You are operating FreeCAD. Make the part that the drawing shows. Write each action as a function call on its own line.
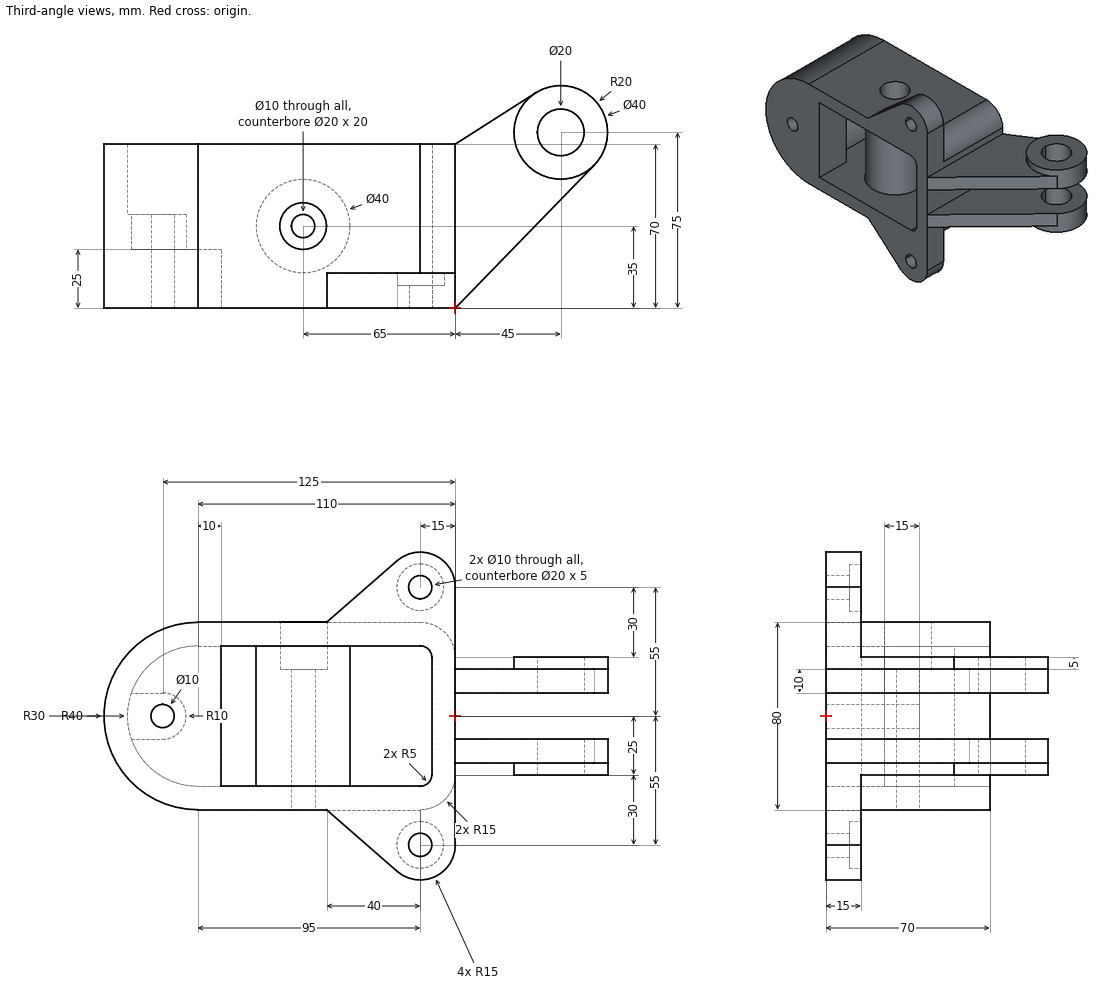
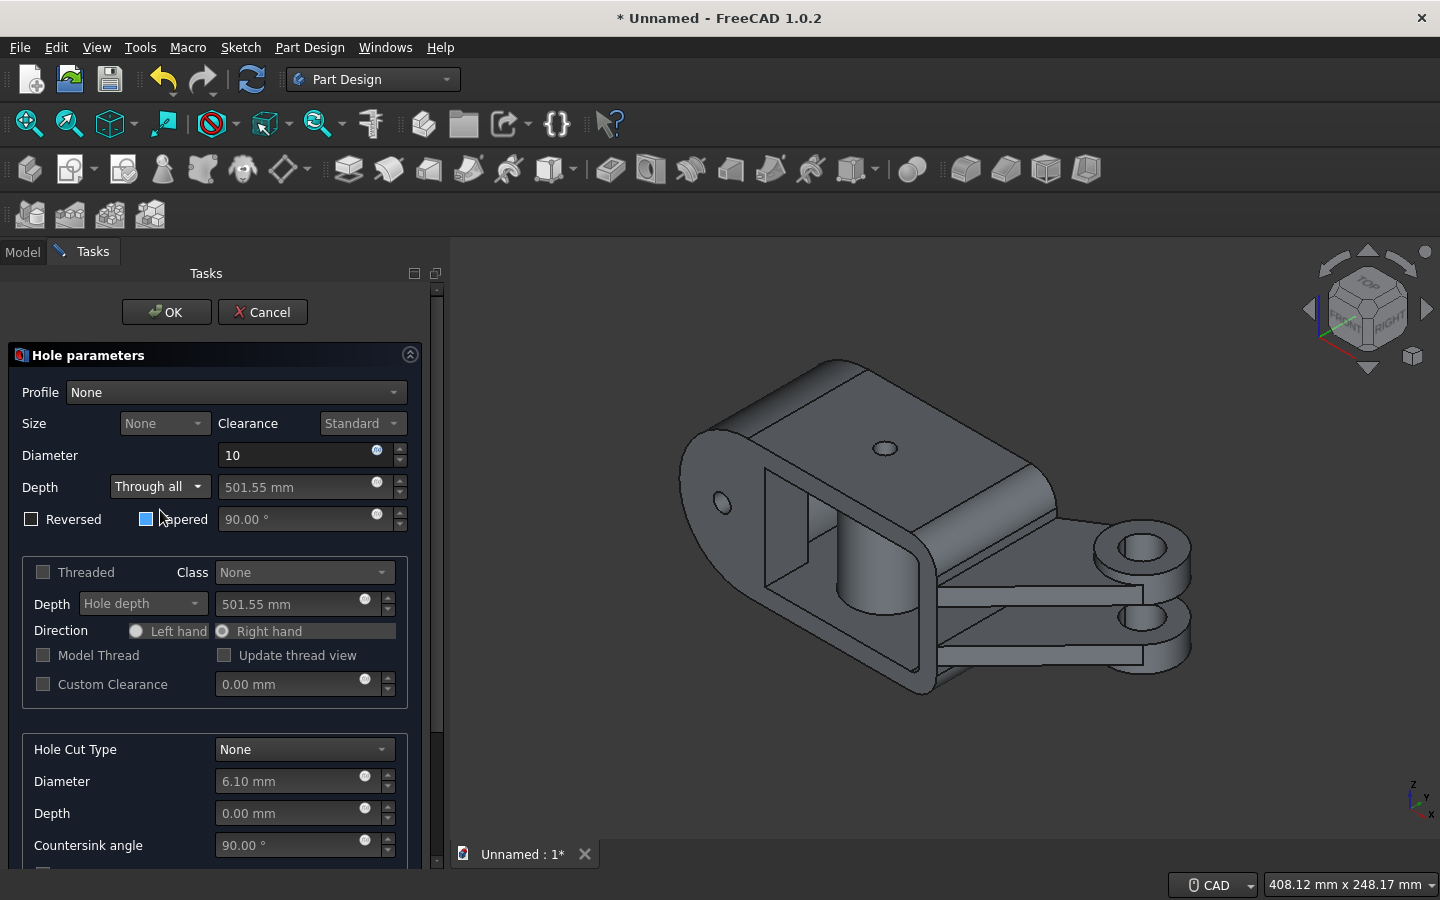
click(306, 750)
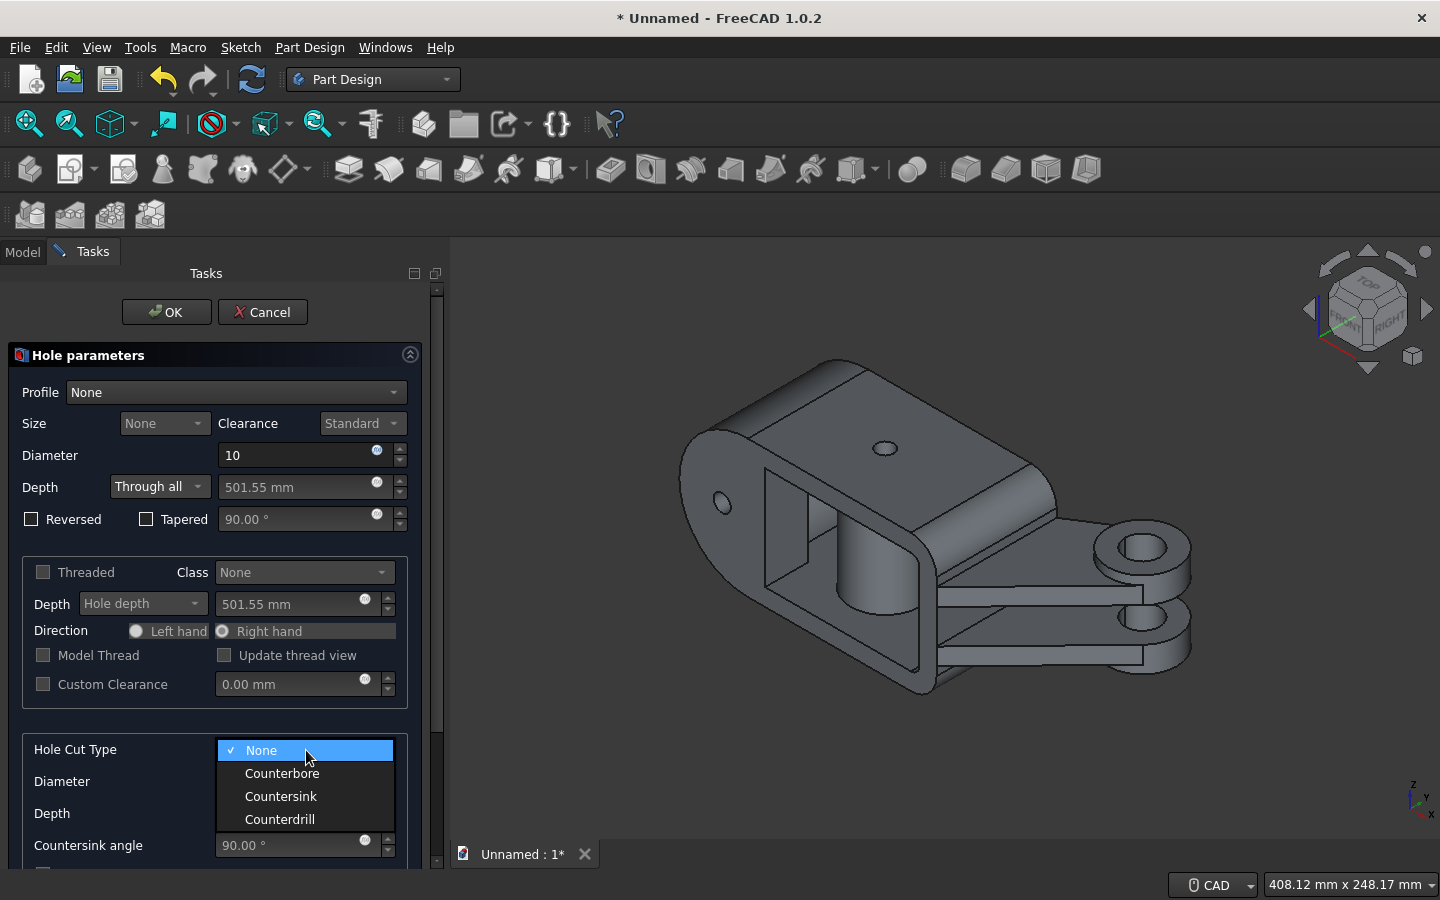
click(304, 774)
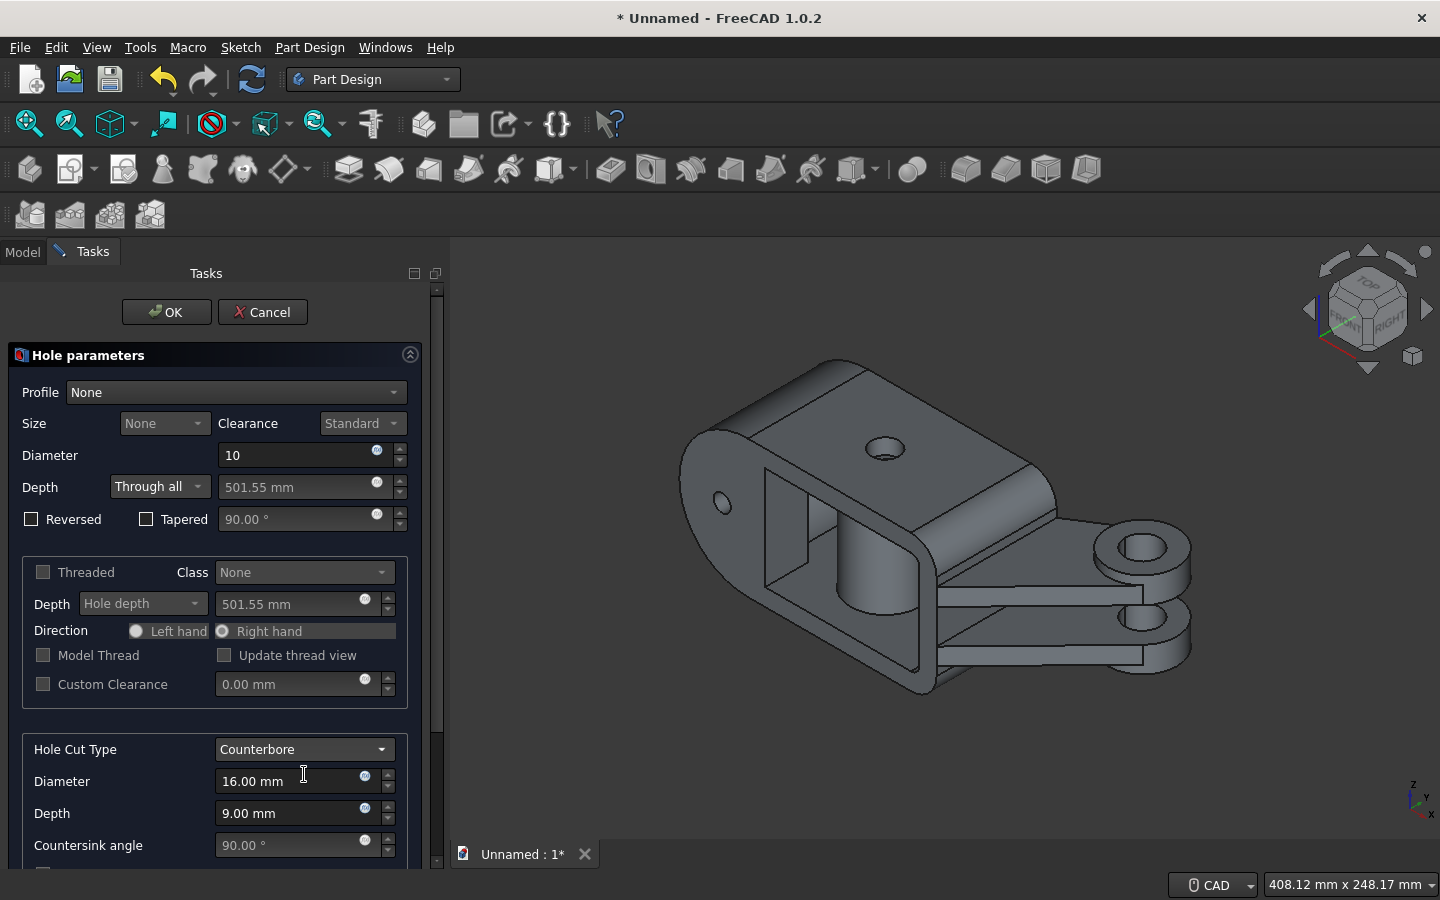
triple_click(298, 781)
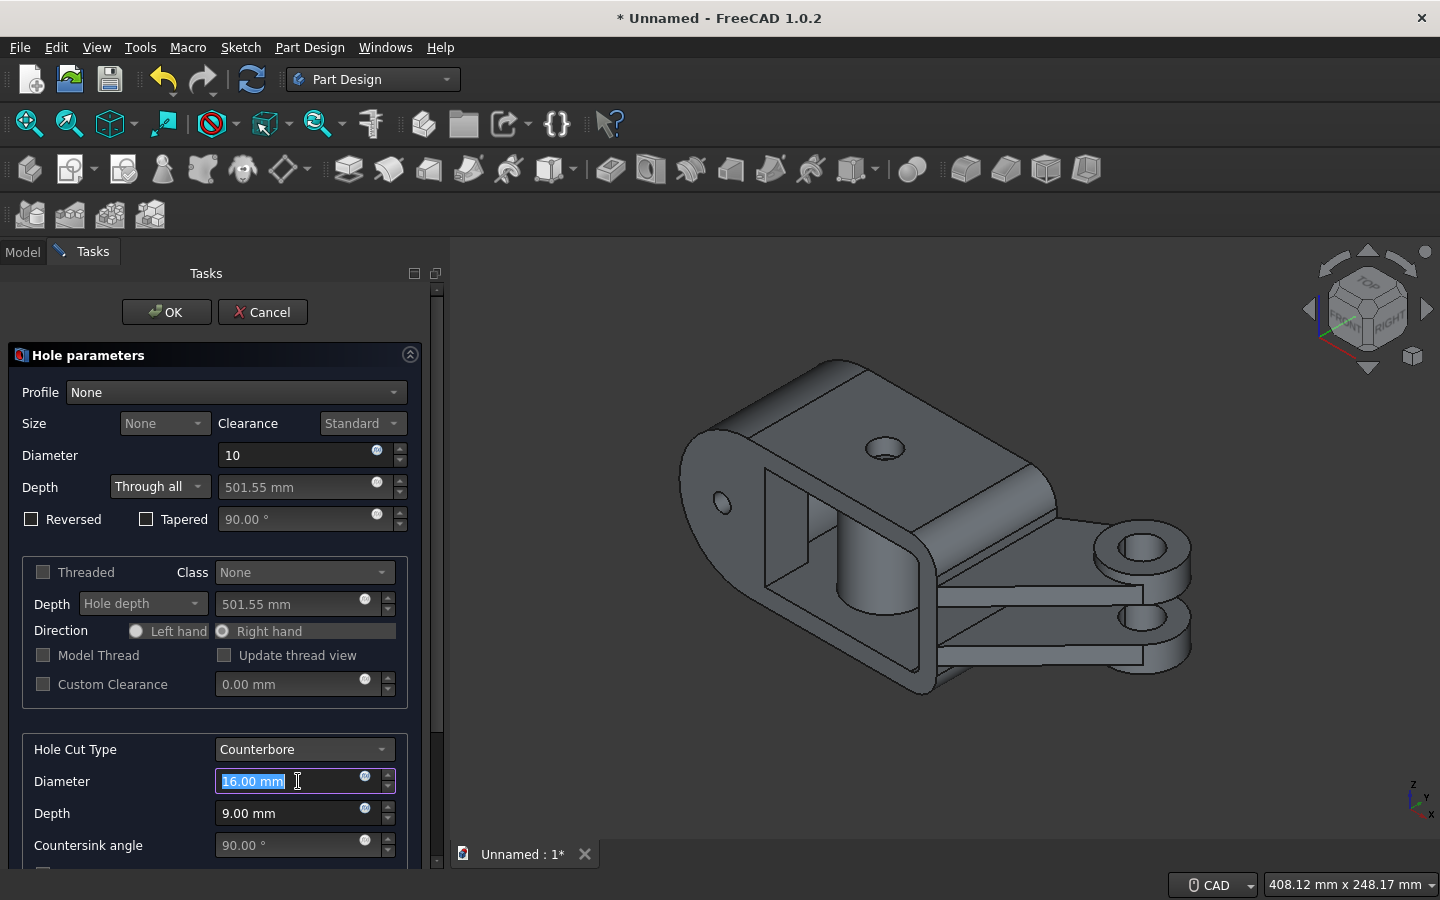
text(20)
key(Tab)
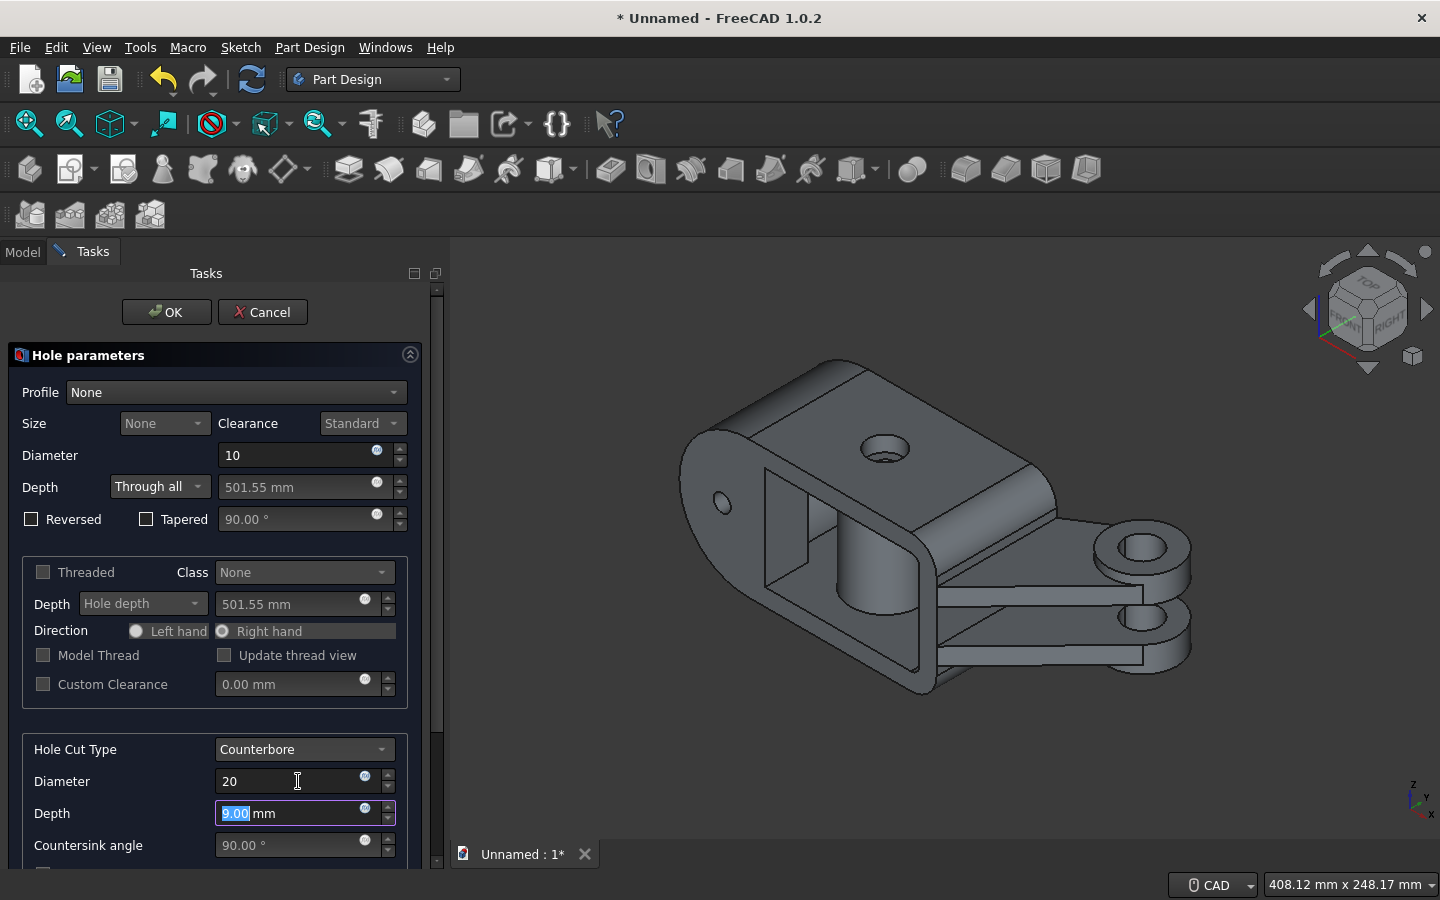
text(20)
key(Tab)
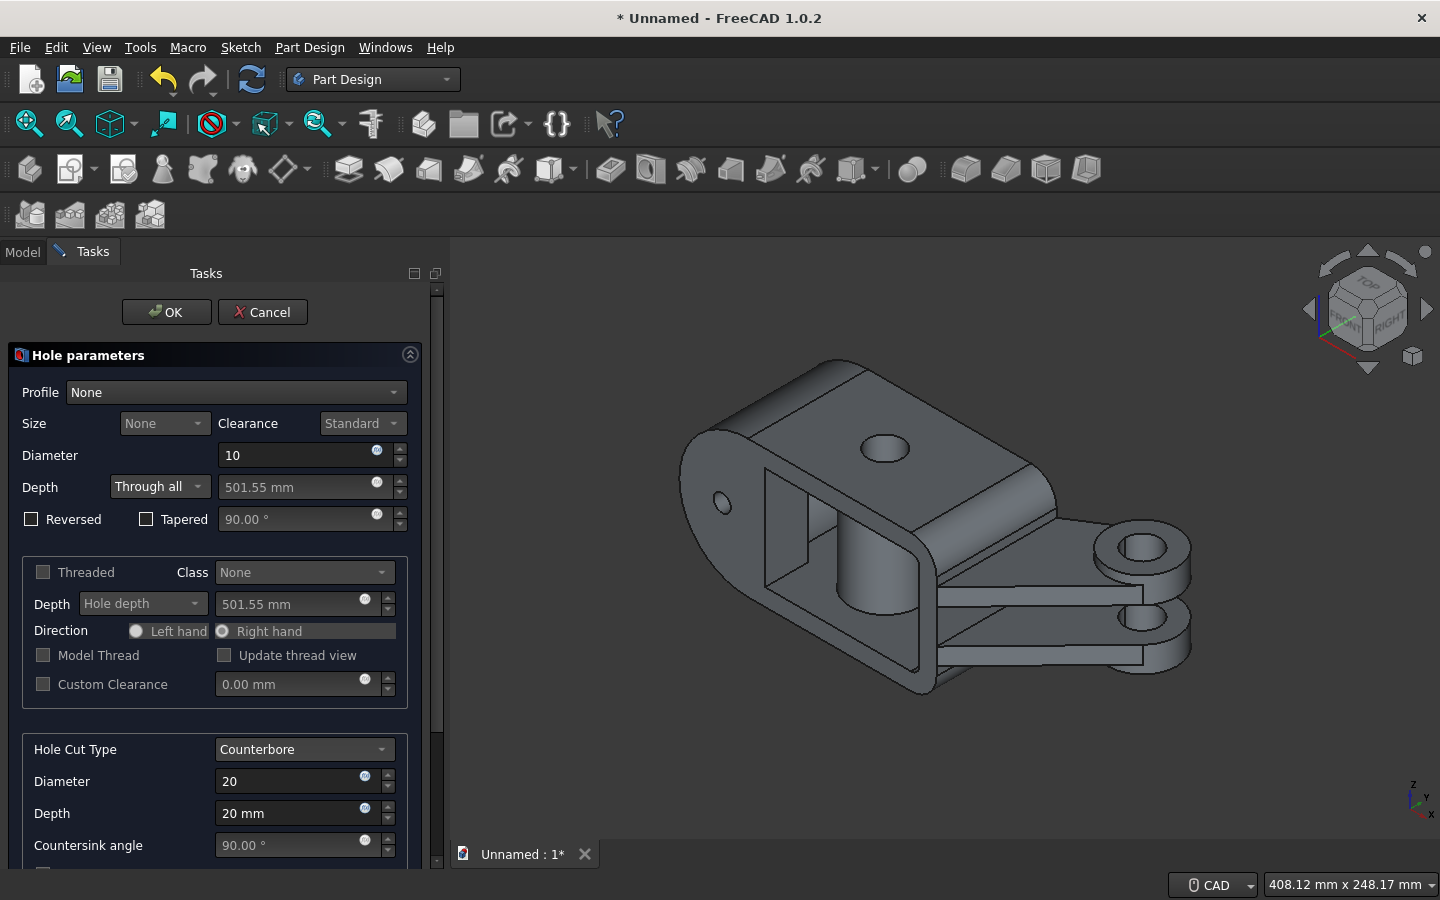
click(167, 312)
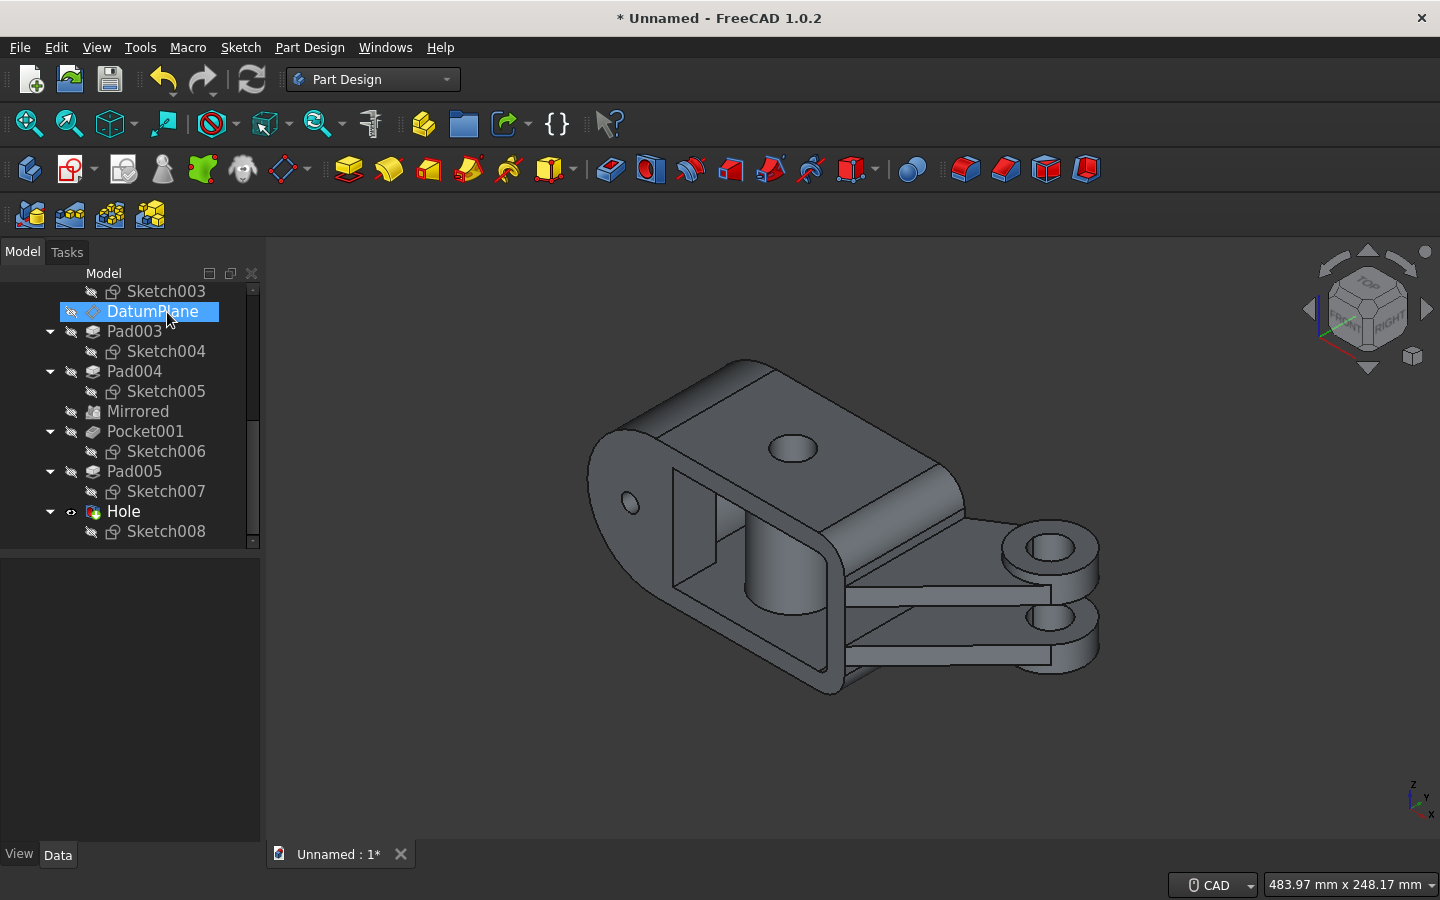
click(642, 464)